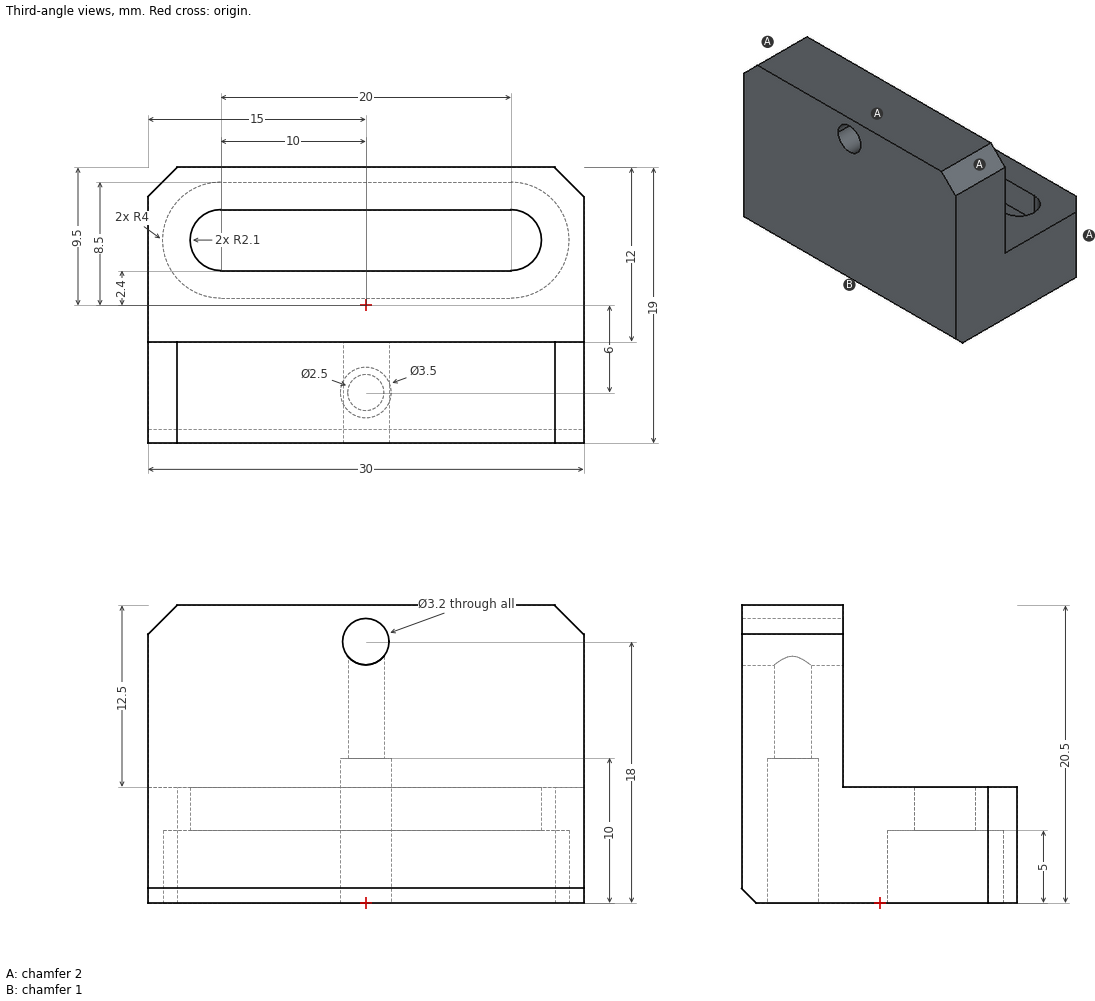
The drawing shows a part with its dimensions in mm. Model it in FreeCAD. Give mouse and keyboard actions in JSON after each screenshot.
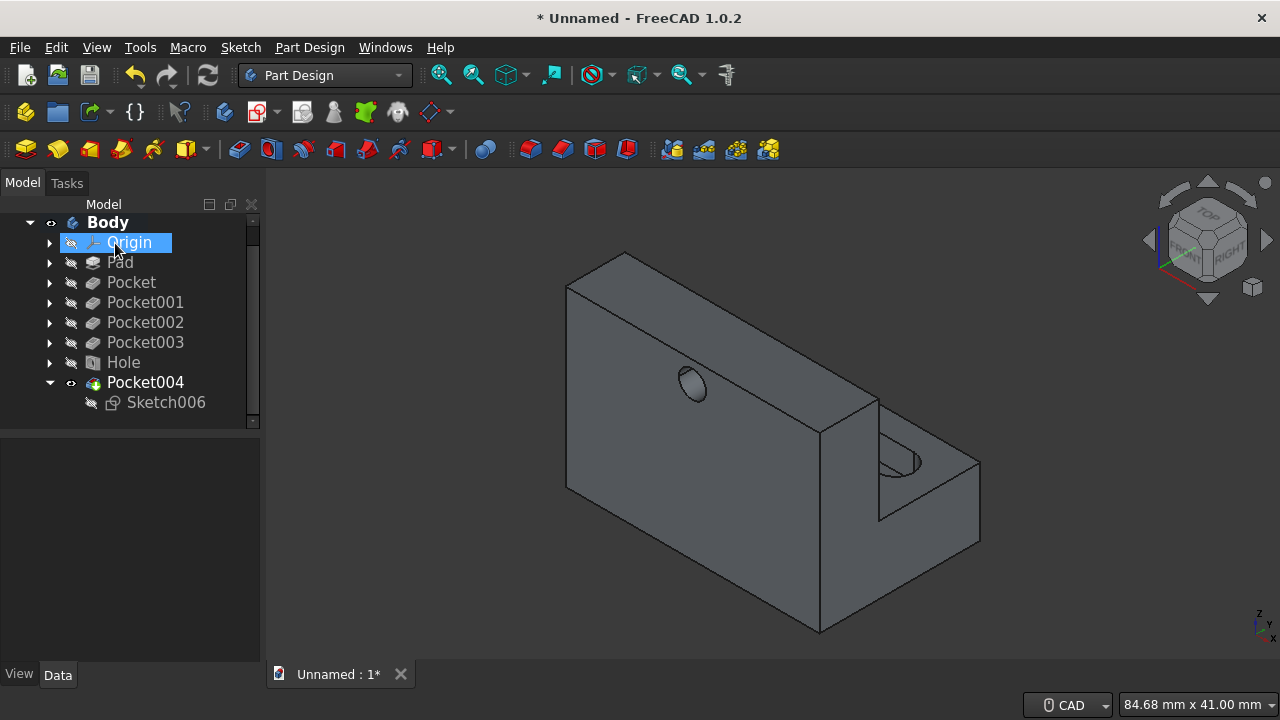
{"action": "left_click", "coordinate": [849, 415]}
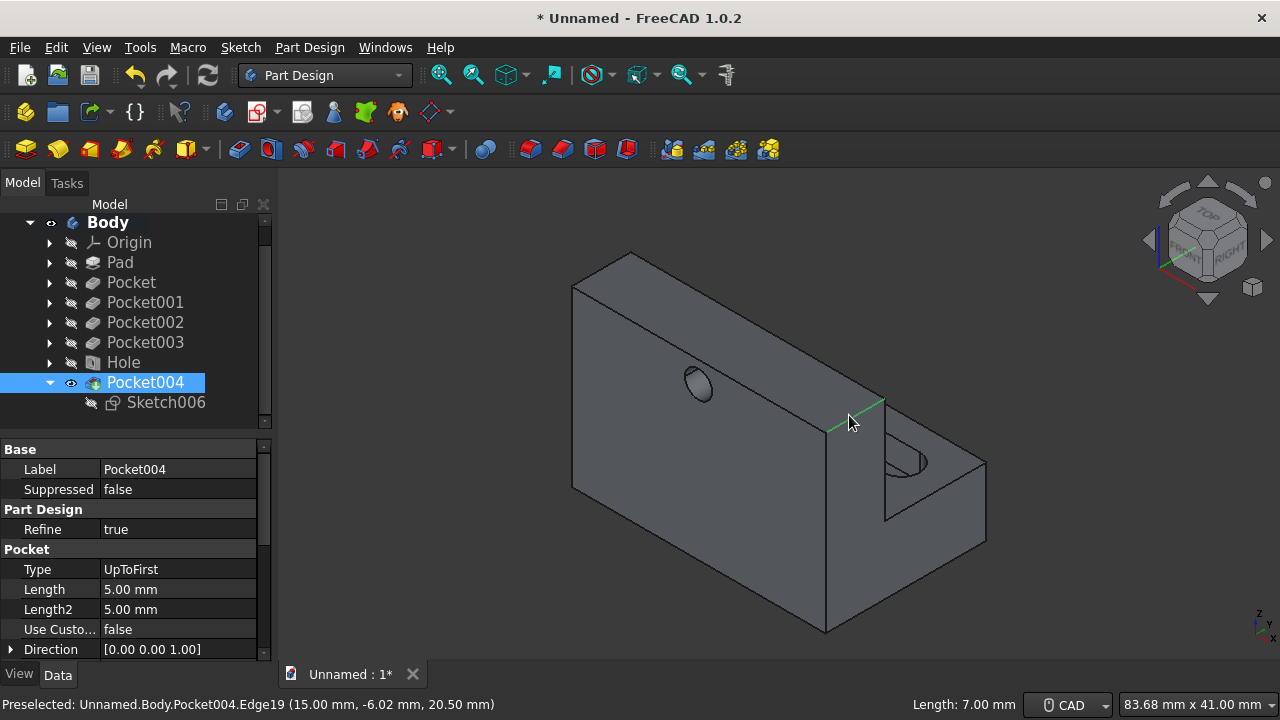
{"action": "key", "text": "2"}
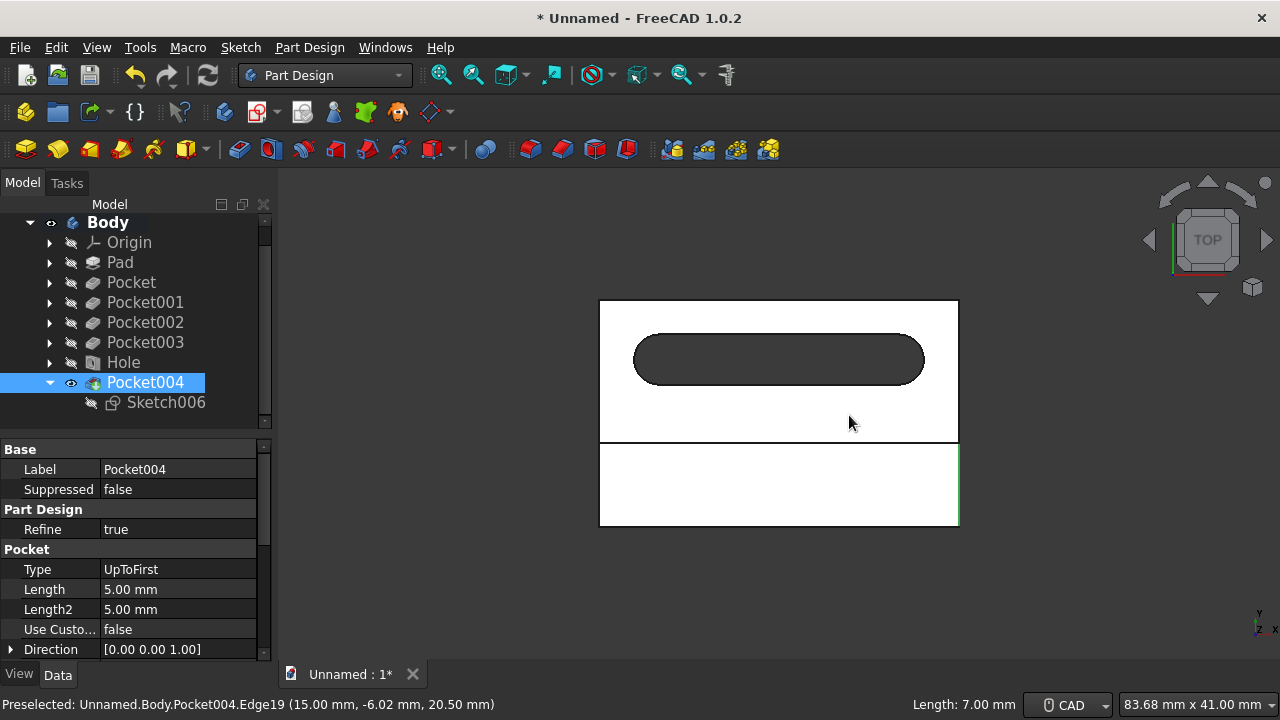
{"action": "left_click", "coordinate": [599, 484], "text": "ctrl"}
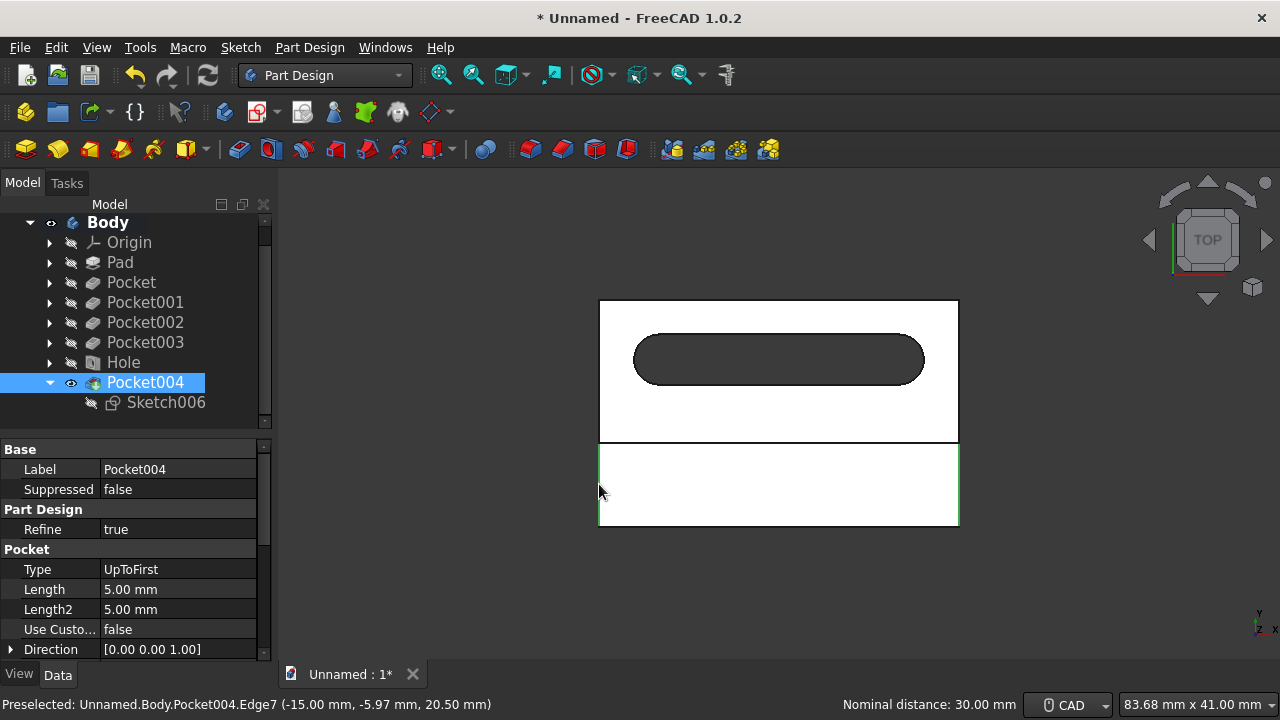
{"action": "key", "text": "1"}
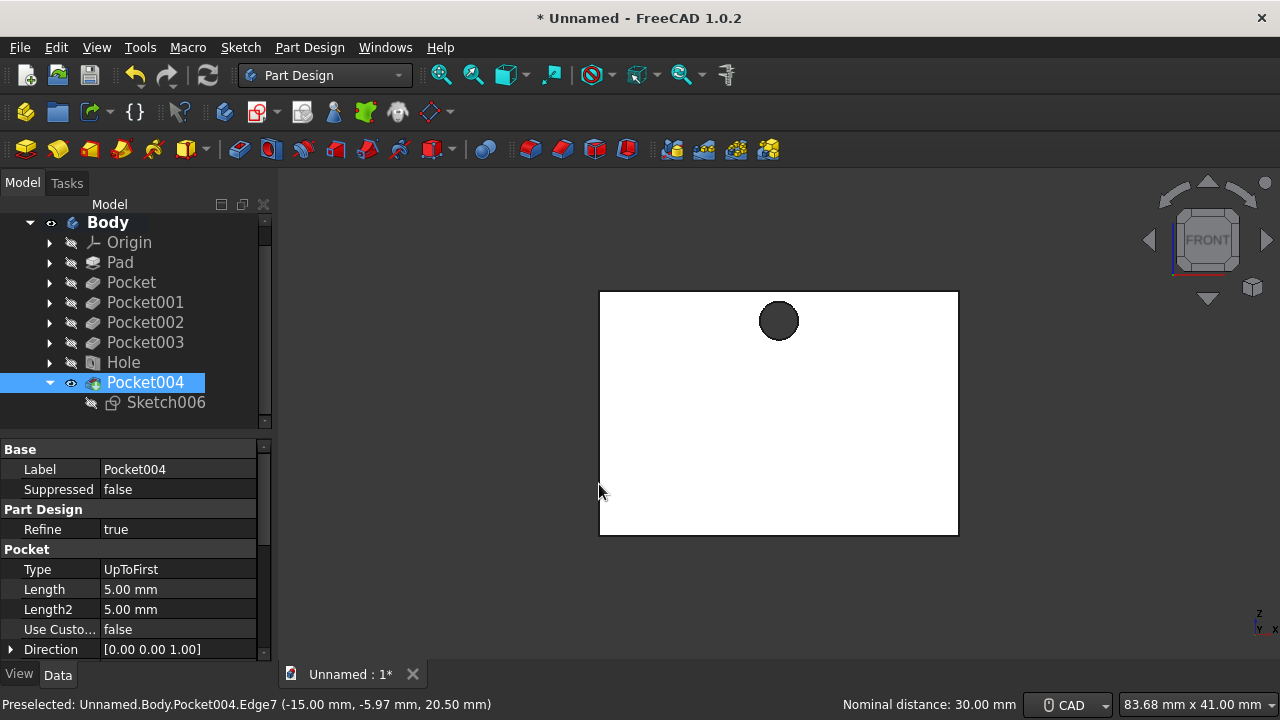
{"action": "key", "text": "3"}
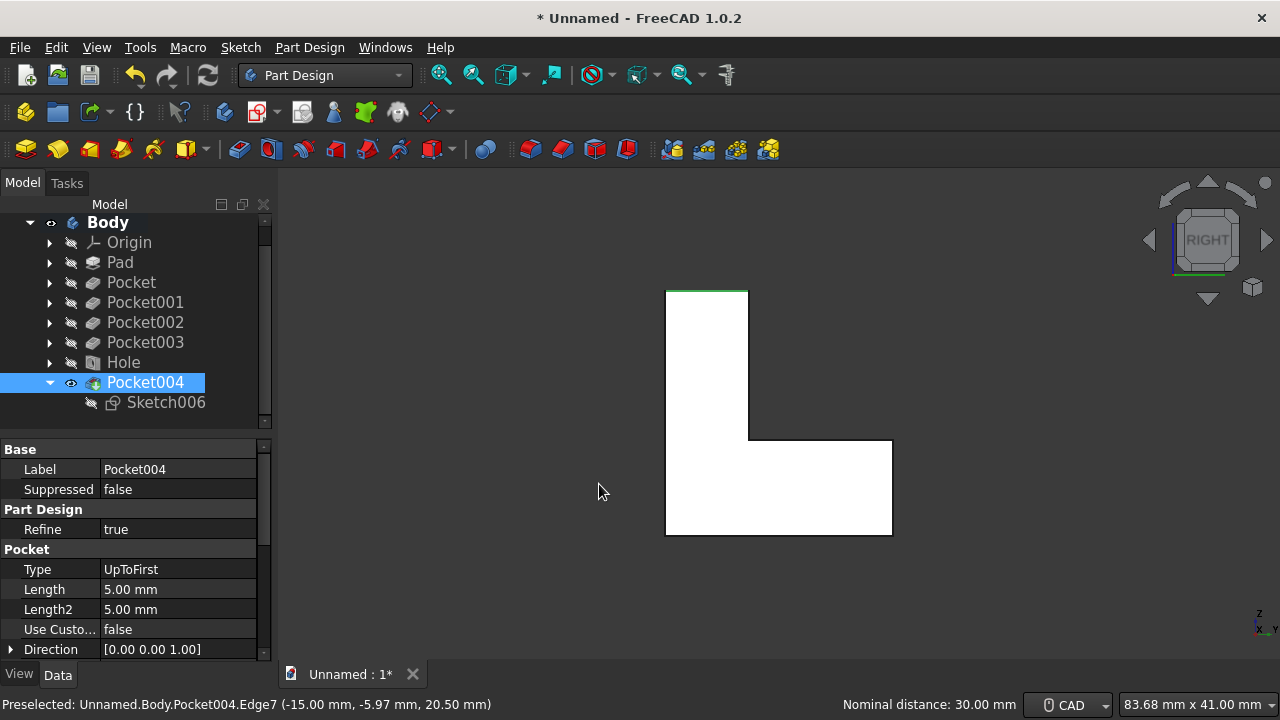
{"action": "left_click", "coordinate": [893, 487], "text": "ctrl"}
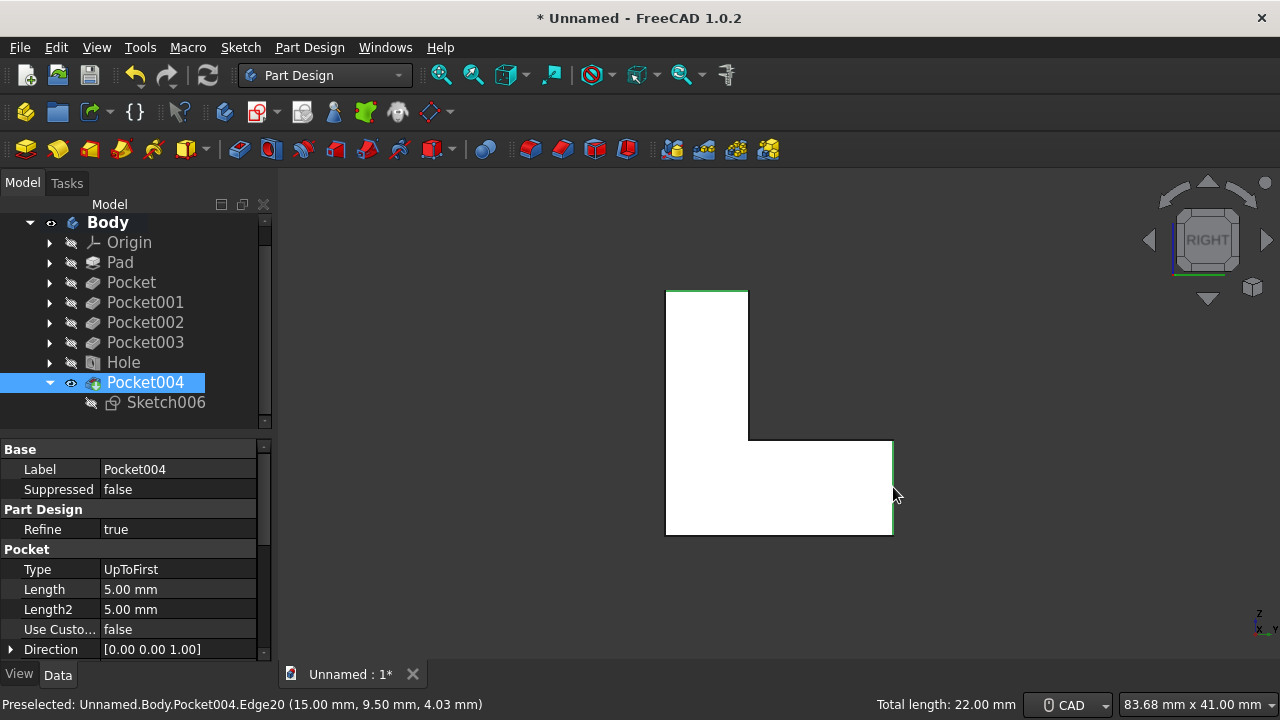
{"action": "key", "text": "5"}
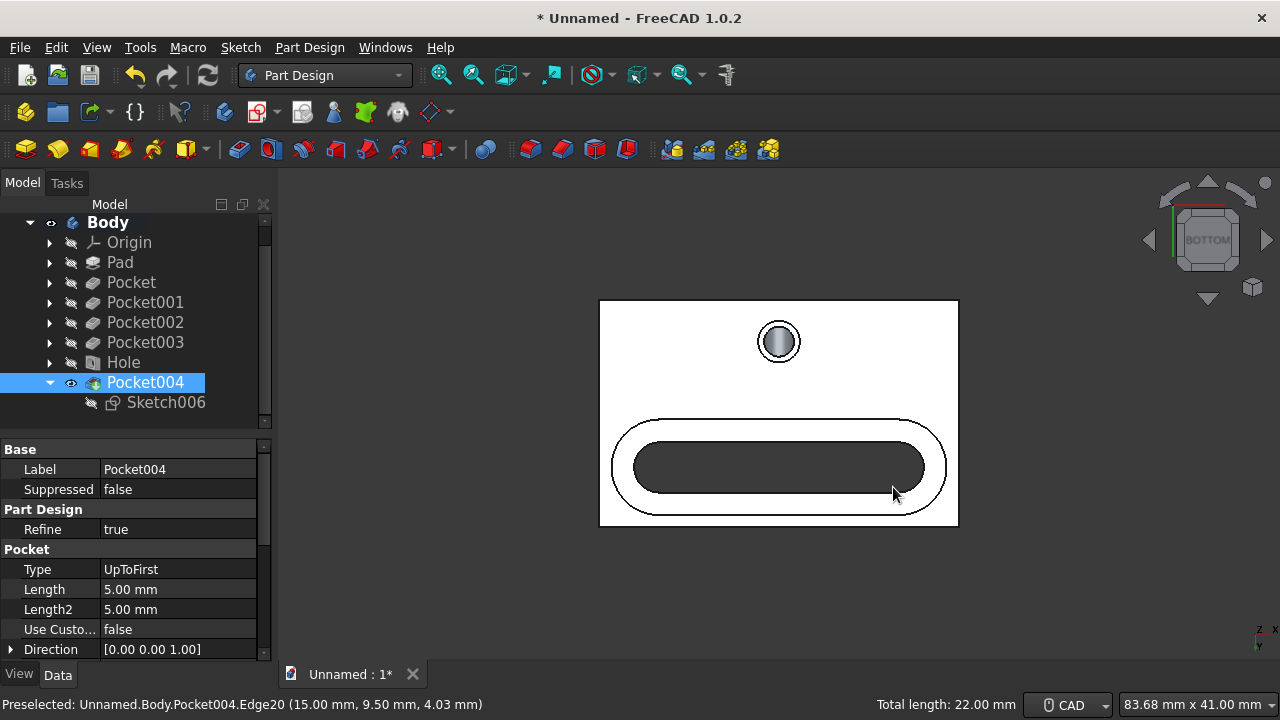
{"action": "key", "text": "4"}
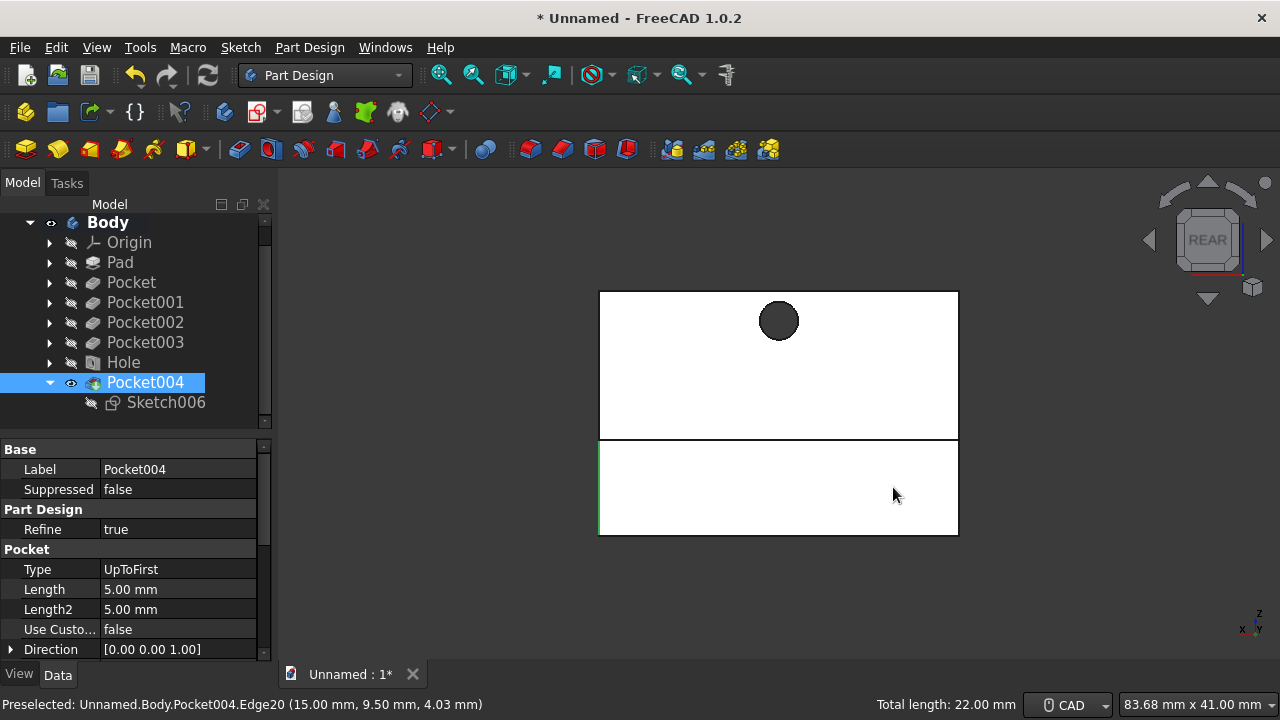
{"action": "left_click", "coordinate": [959, 487], "text": "ctrl"}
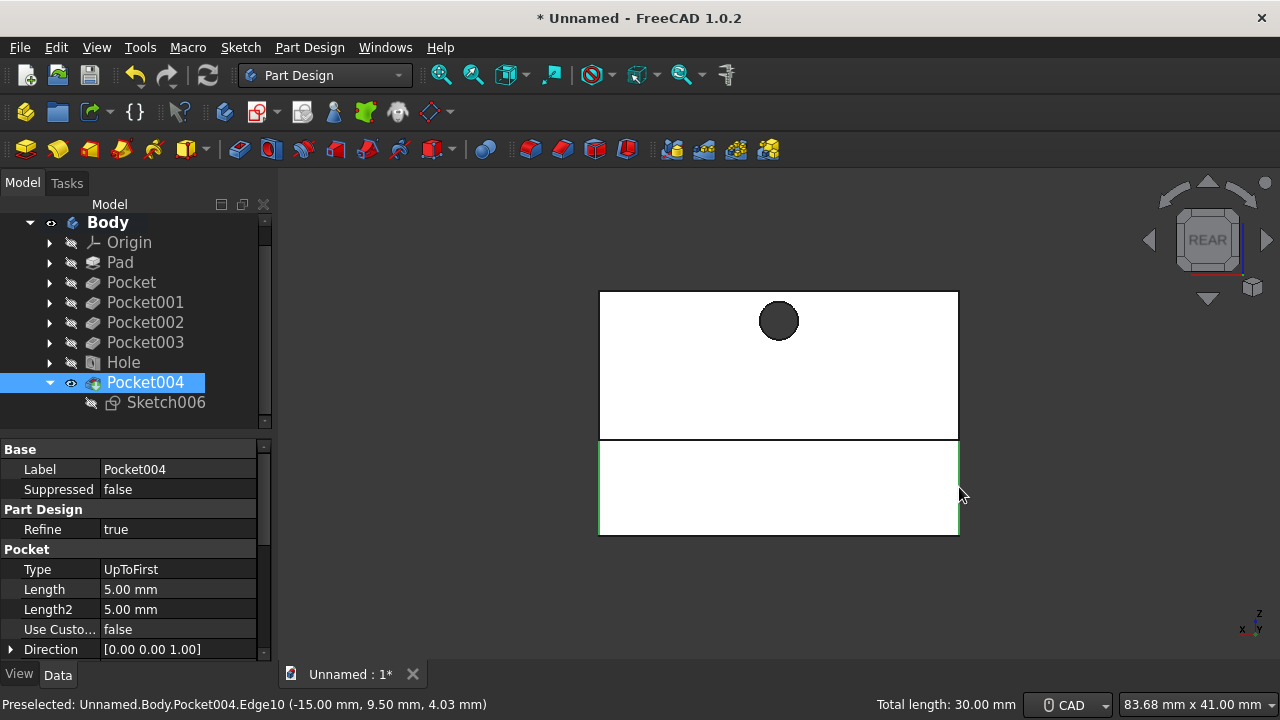
{"action": "left_click", "coordinate": [564, 150]}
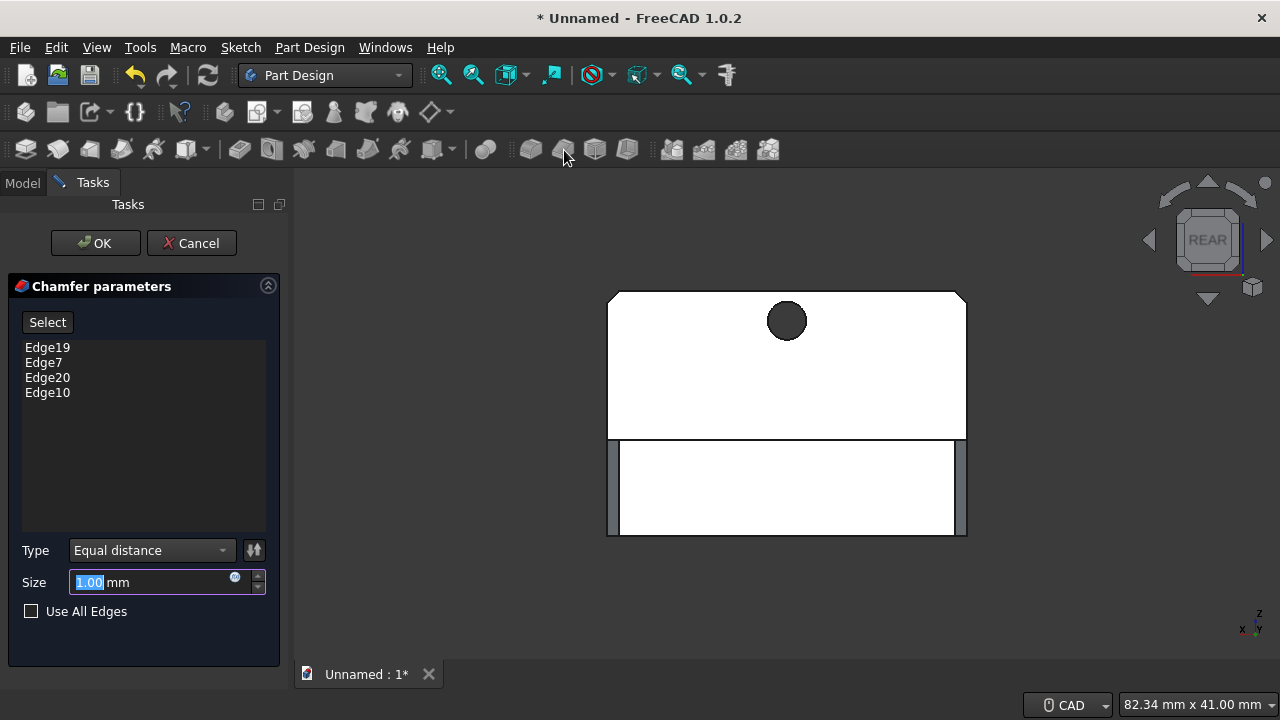
{"action": "type", "text": "2"}
{"action": "key", "text": "Tab"}